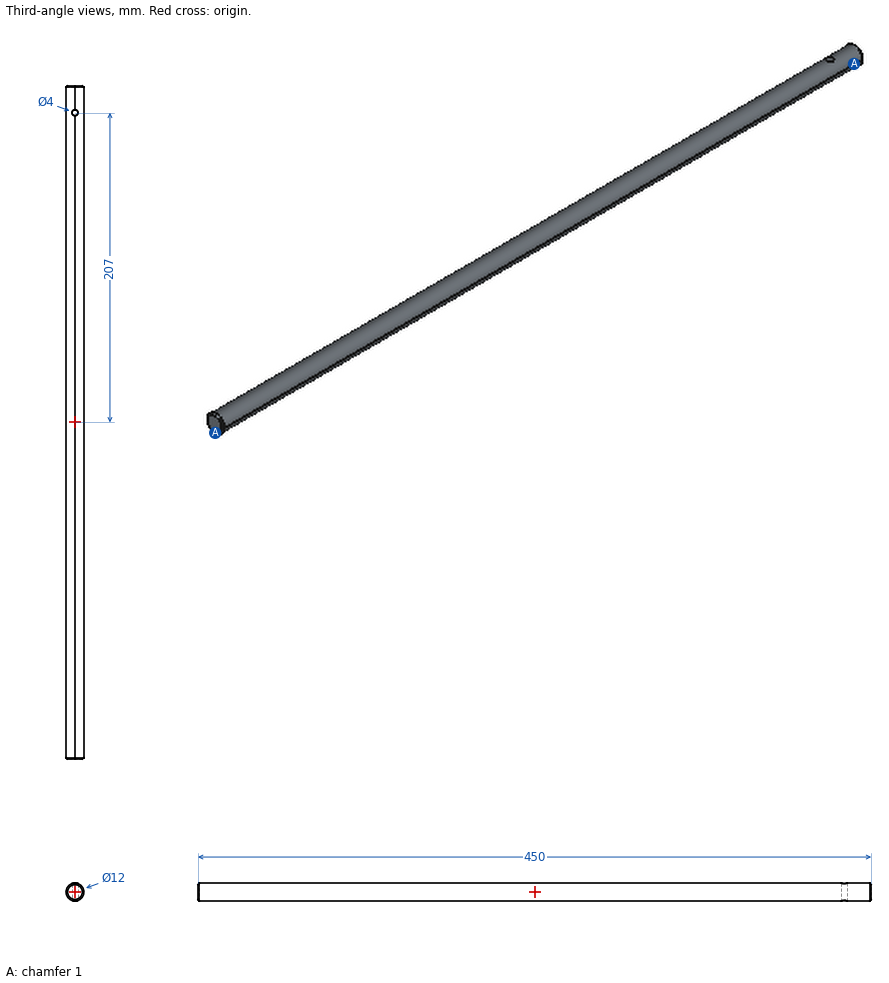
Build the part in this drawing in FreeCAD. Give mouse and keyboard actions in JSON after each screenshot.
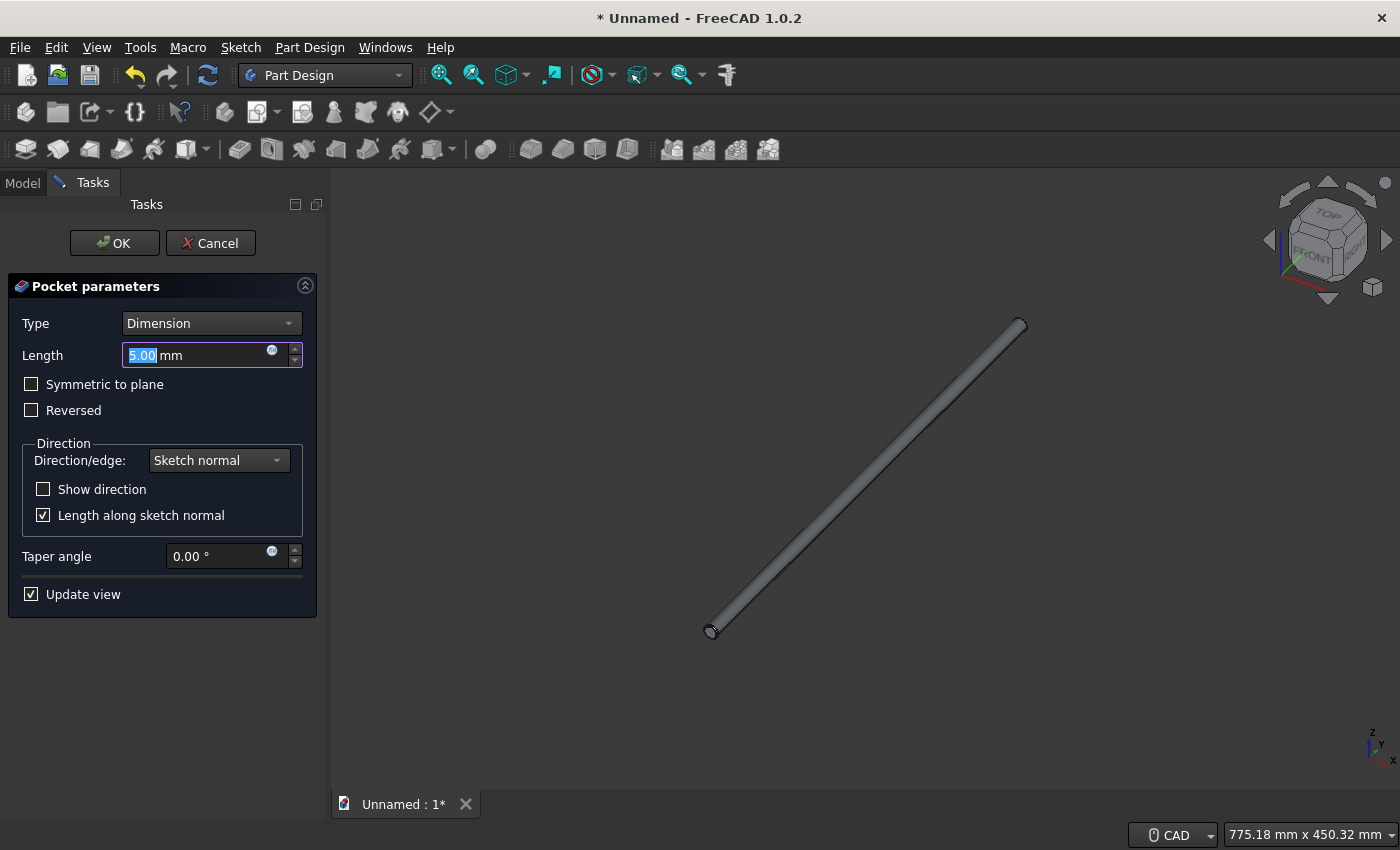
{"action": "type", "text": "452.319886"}
{"action": "key", "text": "Tab"}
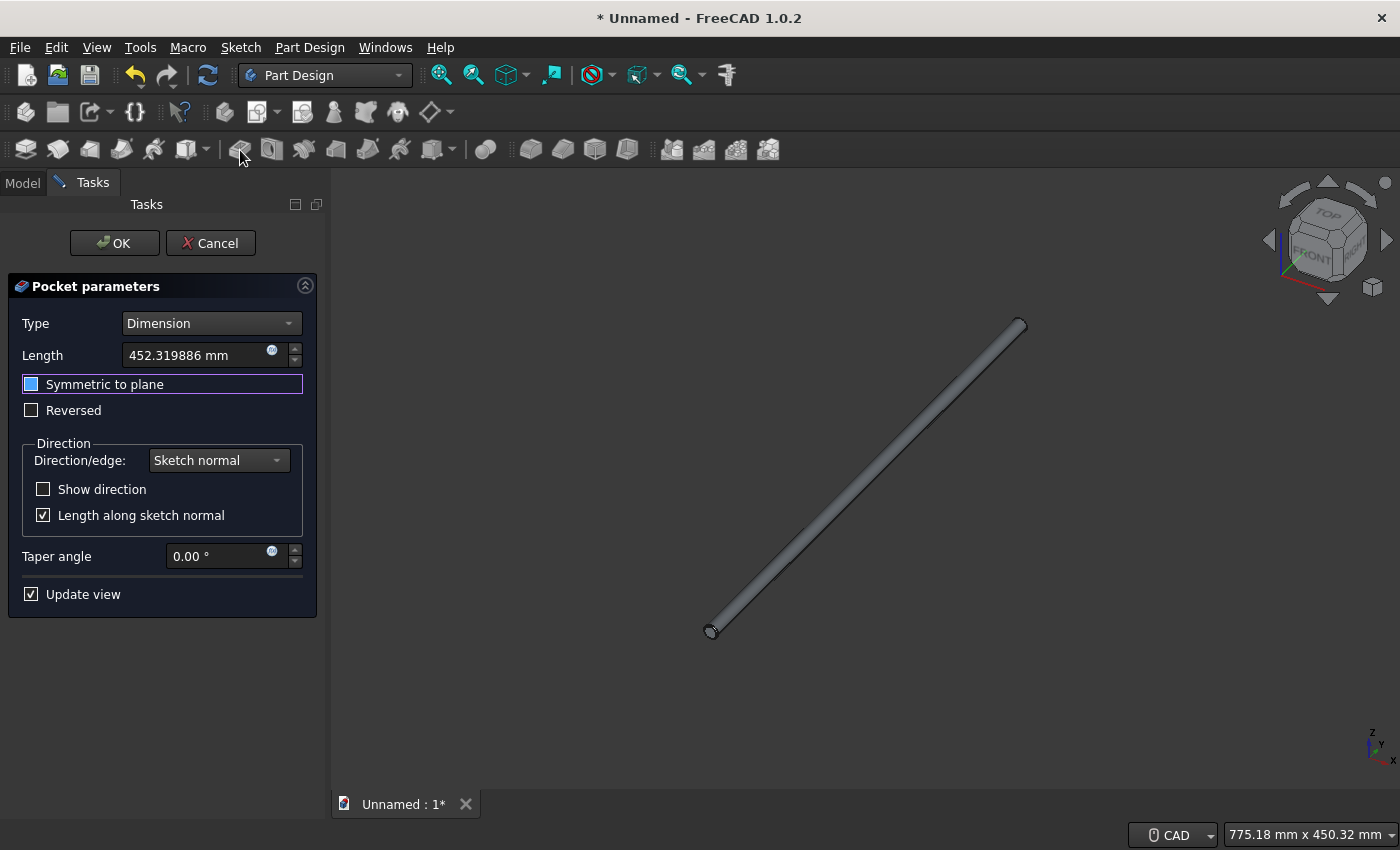
{"action": "left_click", "coordinate": [30, 384]}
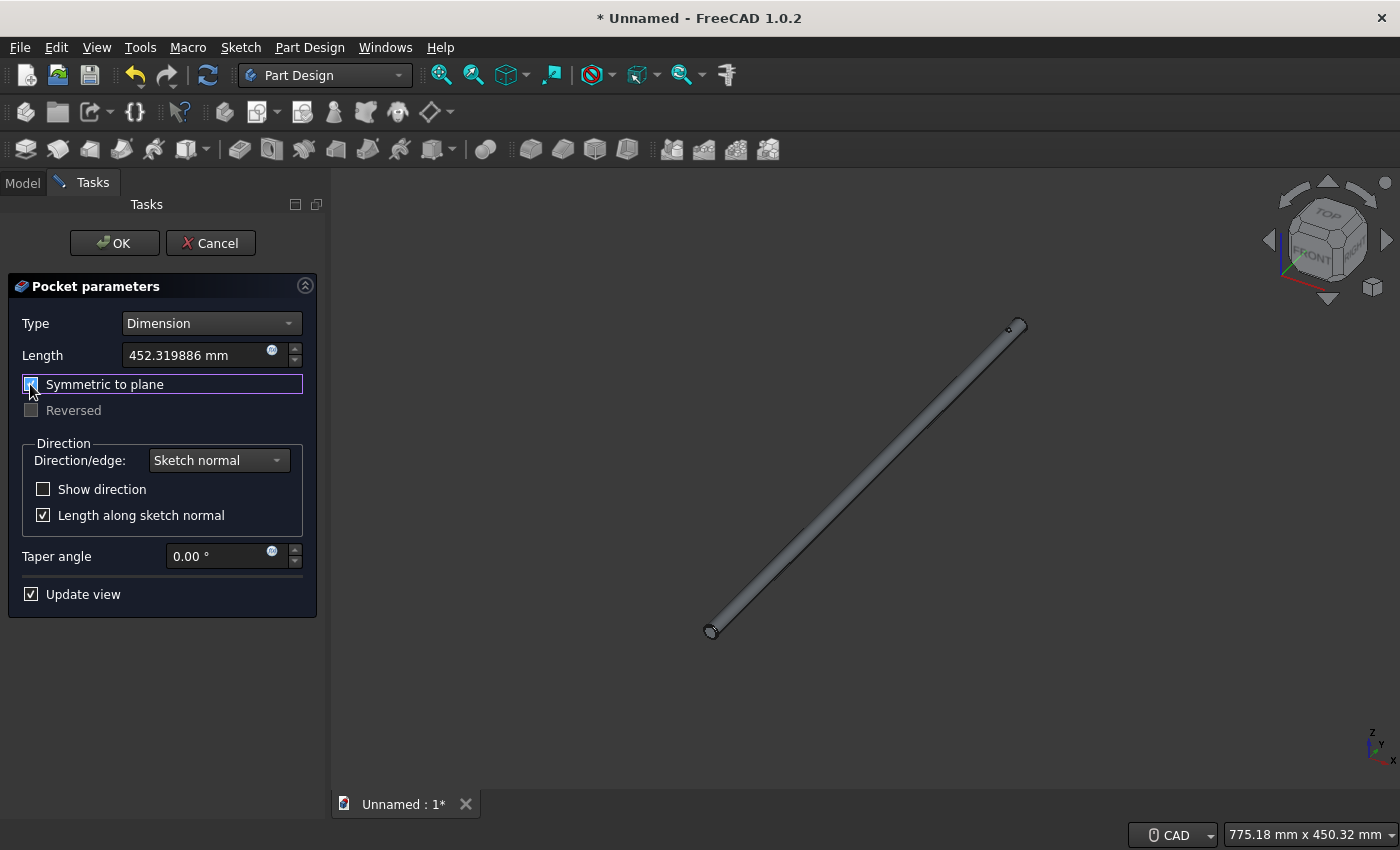
{"action": "left_click", "coordinate": [115, 243]}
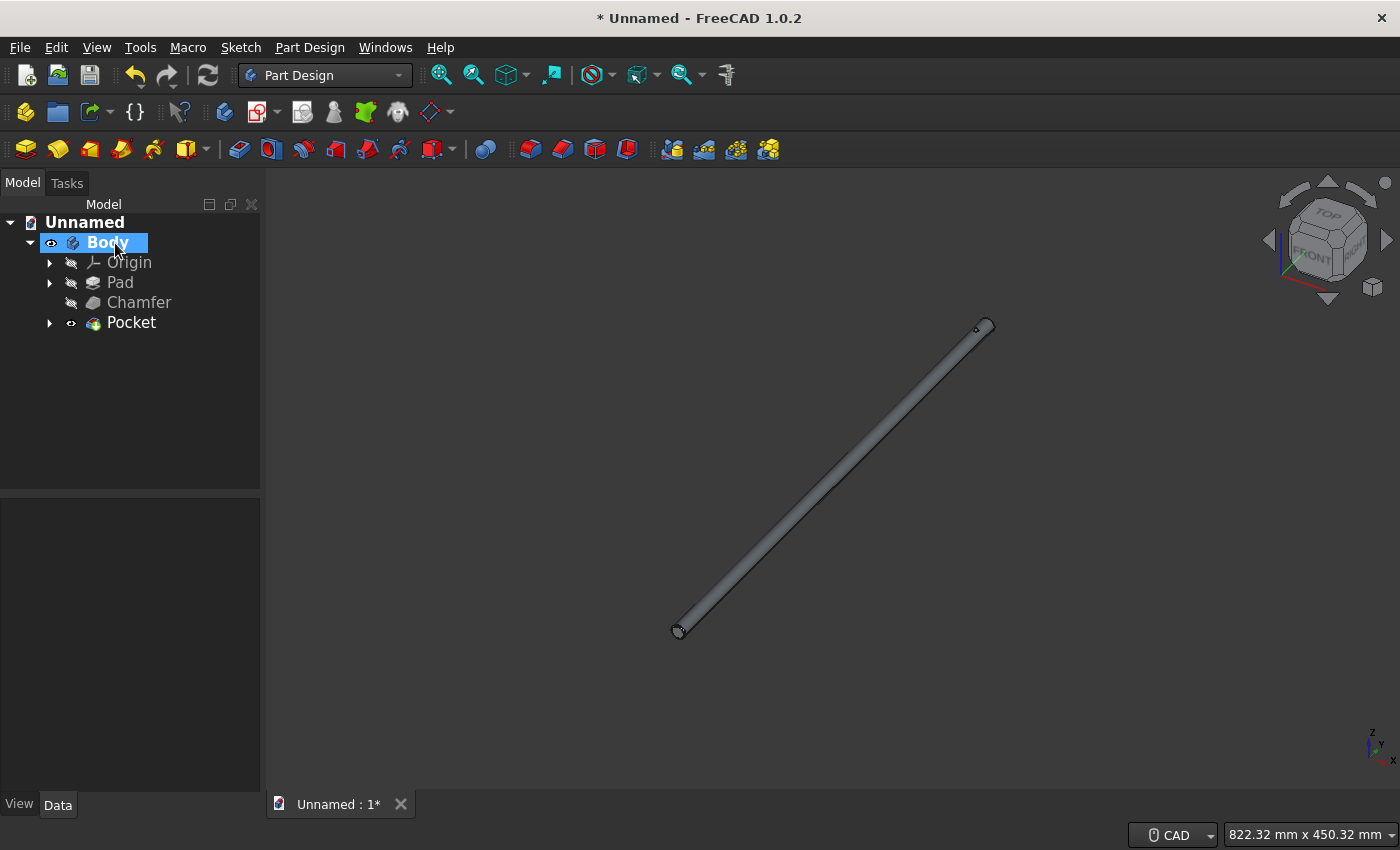
{"action": "key", "text": "0"}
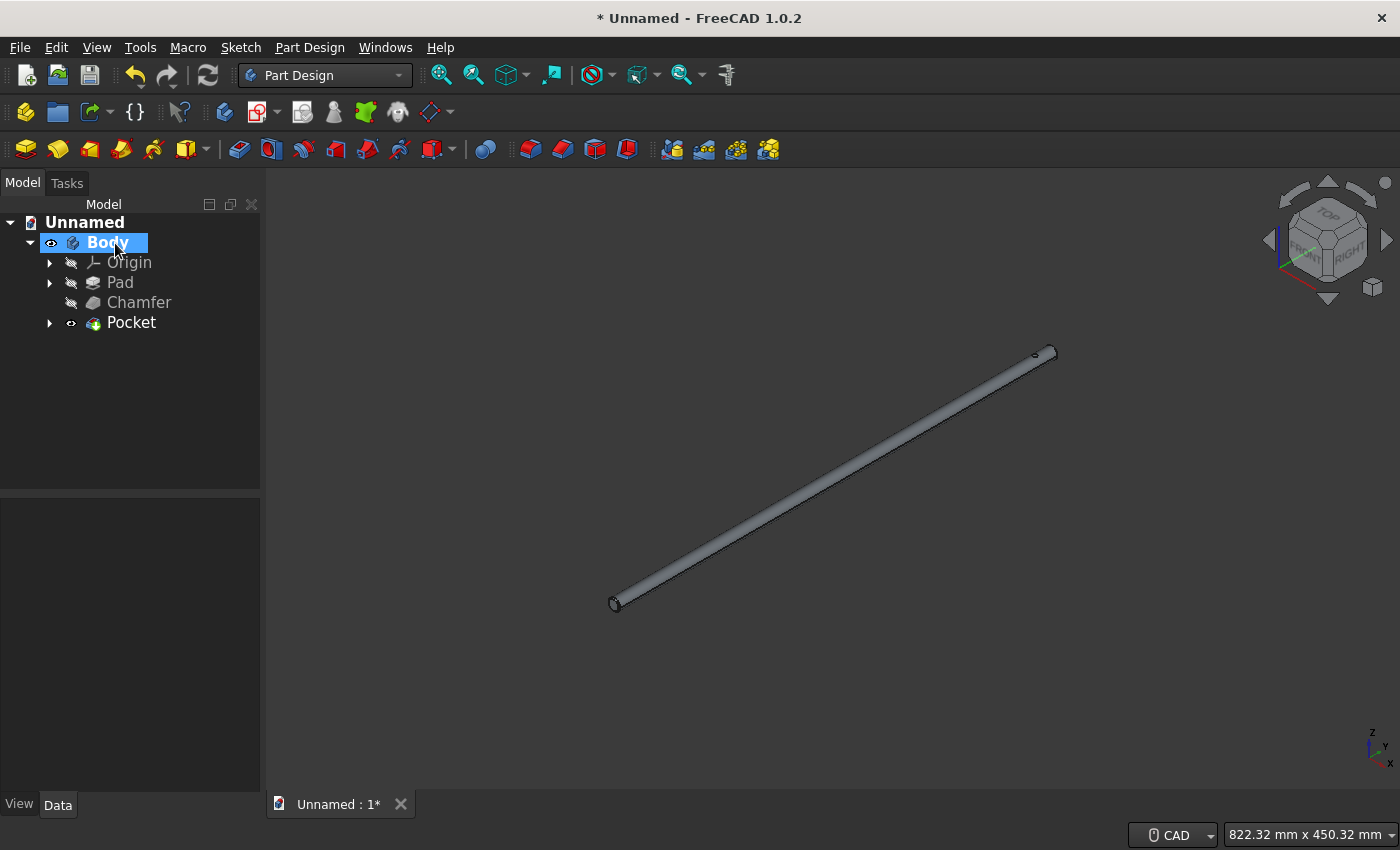
{"action": "key", "text": "v f"}